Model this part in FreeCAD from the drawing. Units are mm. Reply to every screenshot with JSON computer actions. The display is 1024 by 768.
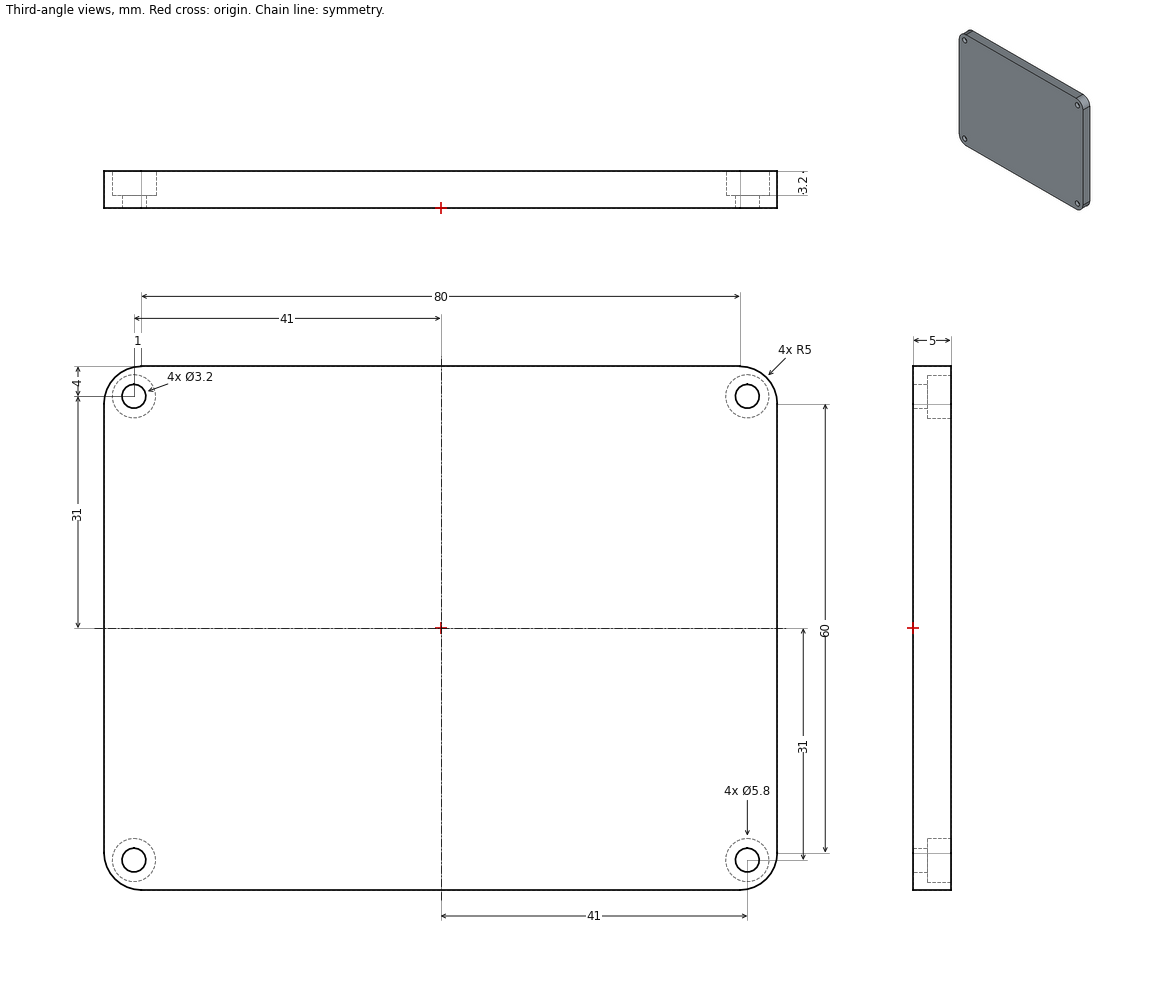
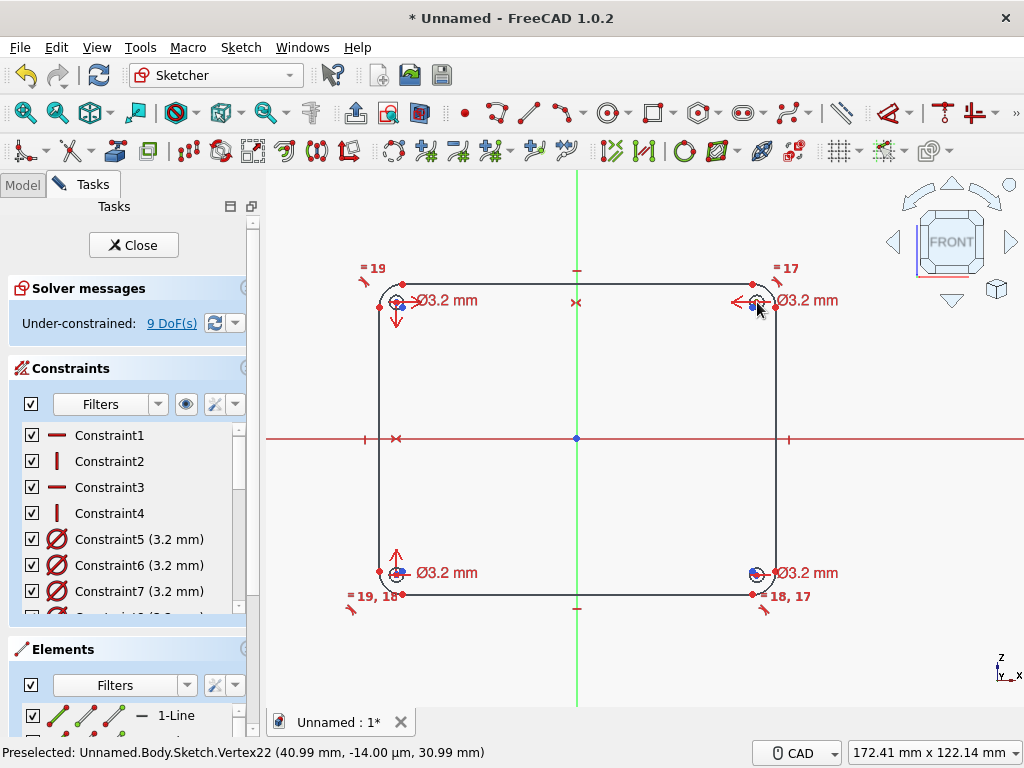
{"action": "scroll", "coordinate": [757, 575], "scroll_direction": "up", "scroll_amount": 4}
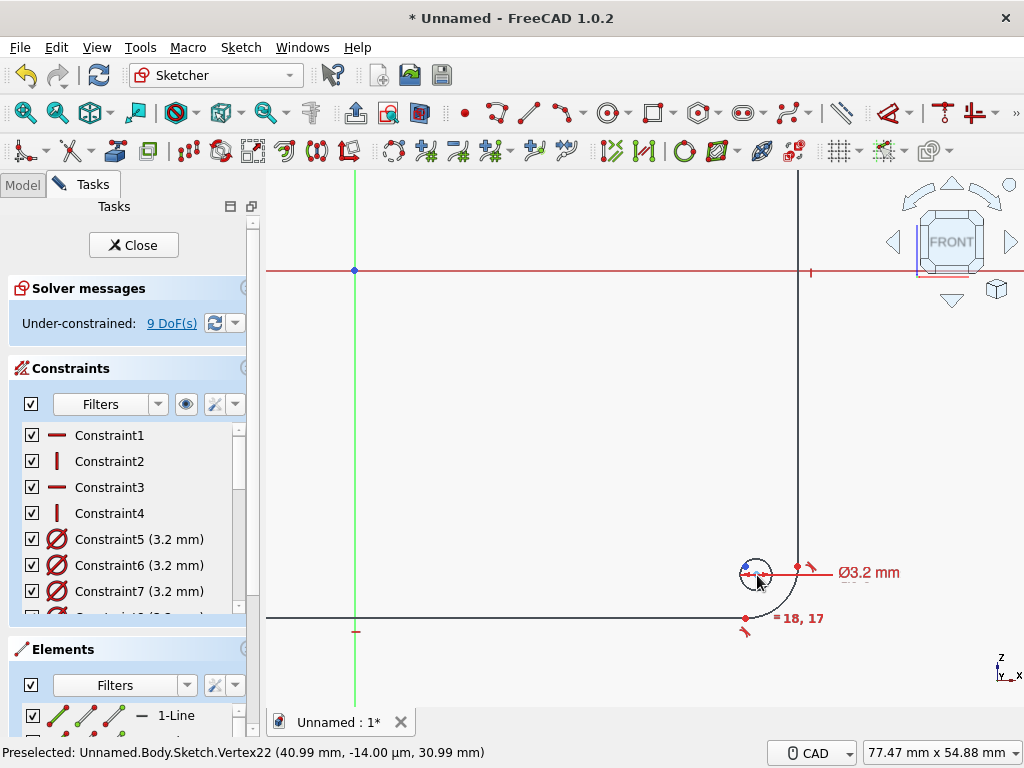
{"action": "left_click", "coordinate": [756, 575]}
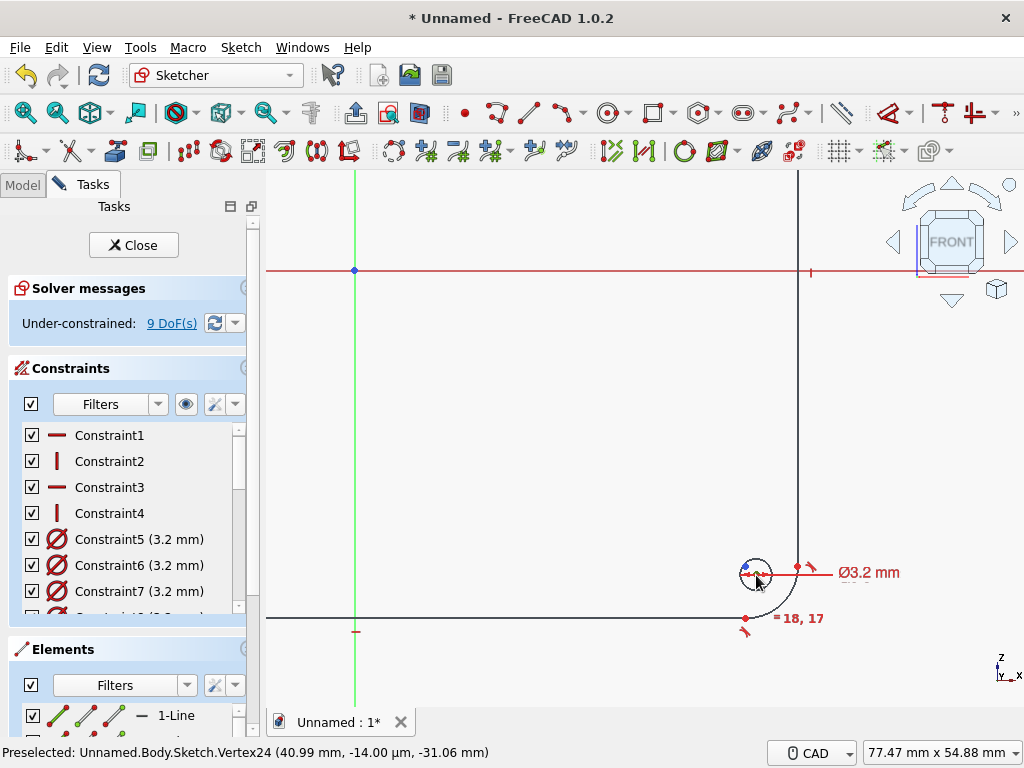
{"action": "left_click", "coordinate": [415, 271]}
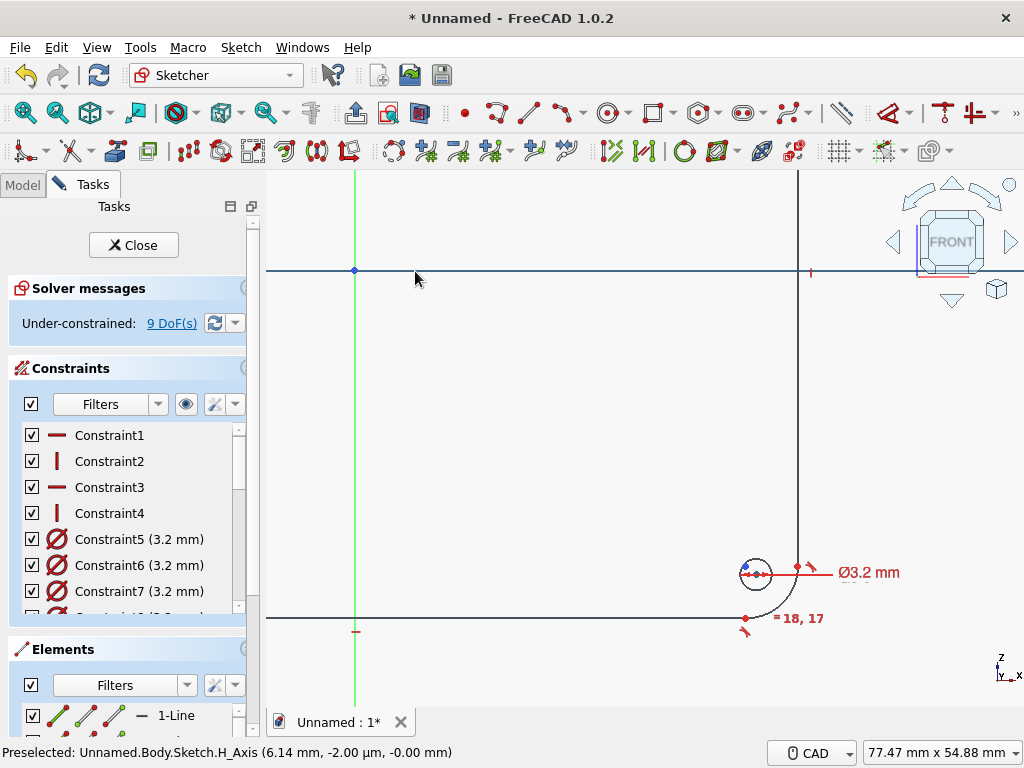
{"action": "key", "text": "s"}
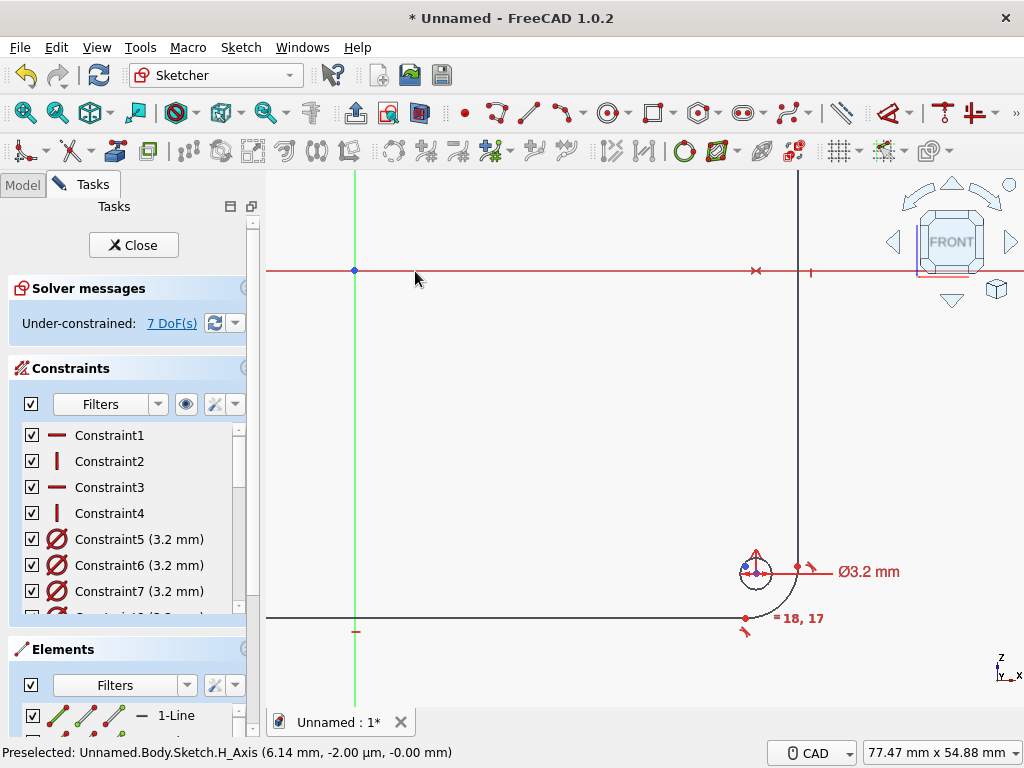
{"action": "scroll", "coordinate": [757, 575], "scroll_direction": "down", "scroll_amount": 4}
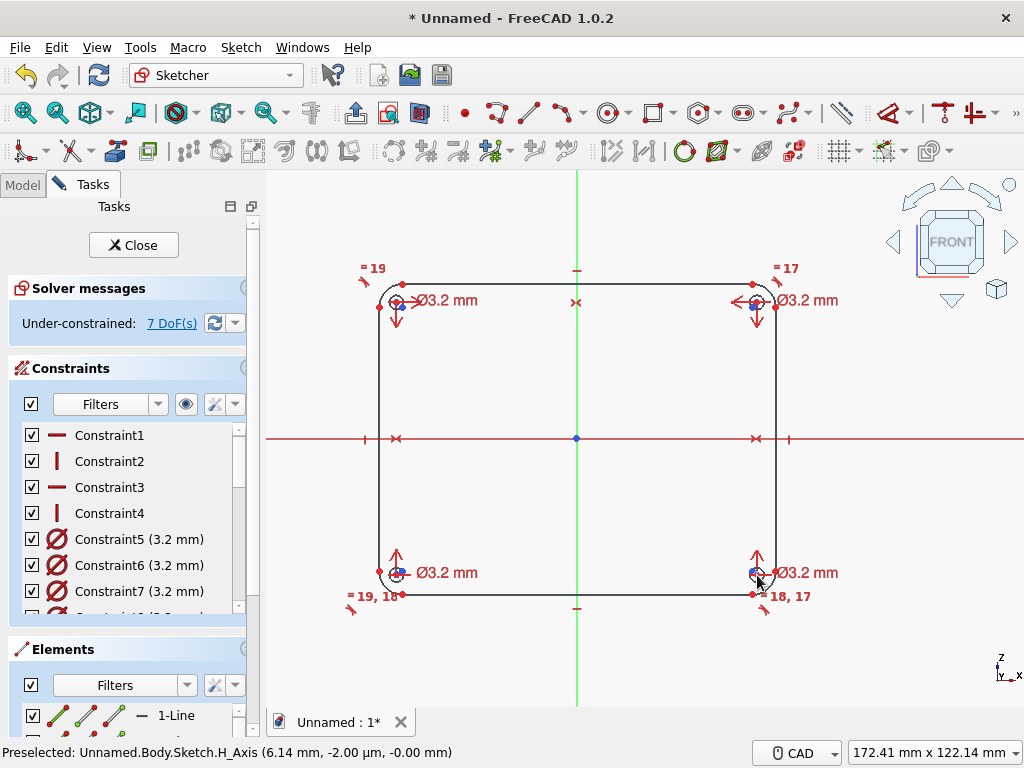
{"action": "scroll", "coordinate": [773, 297], "scroll_direction": "up", "scroll_amount": 3}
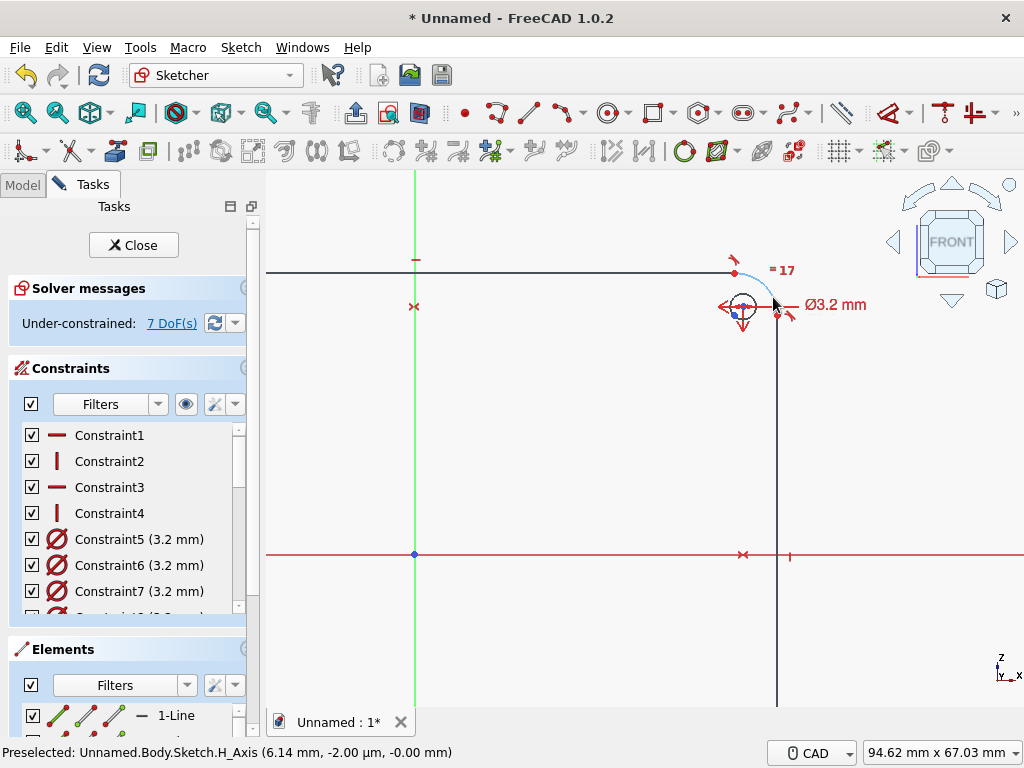
{"action": "left_click", "coordinate": [773, 297]}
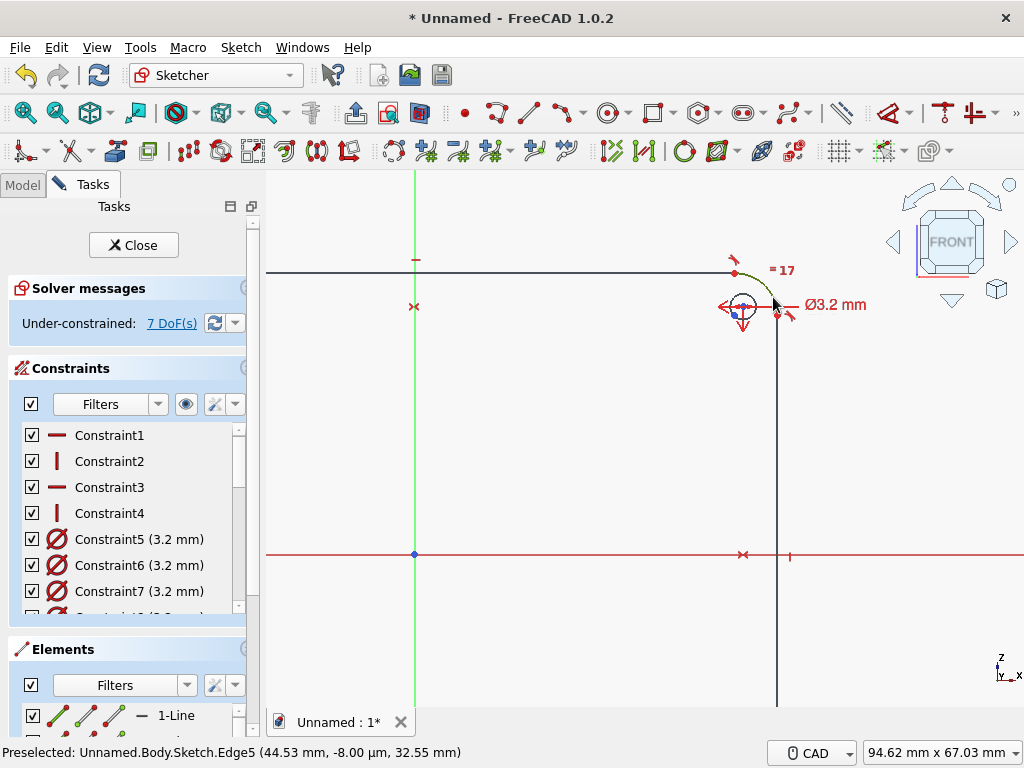
{"action": "key", "text": "k r"}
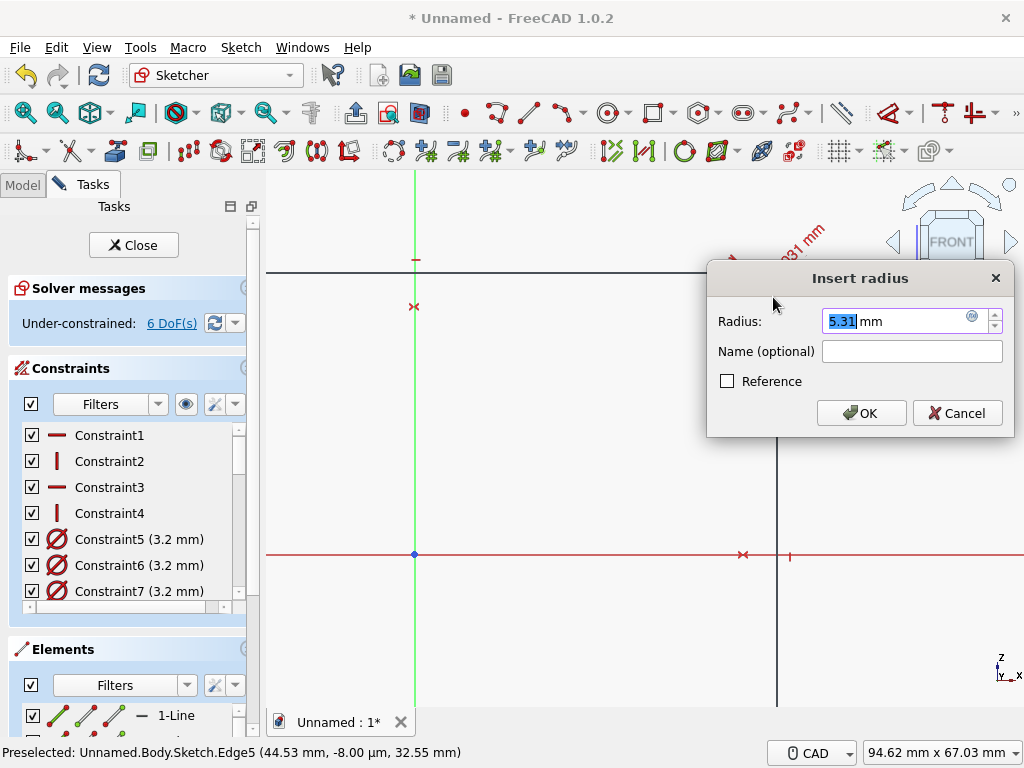
{"action": "type", "text": "5"}
{"action": "key", "text": "Return"}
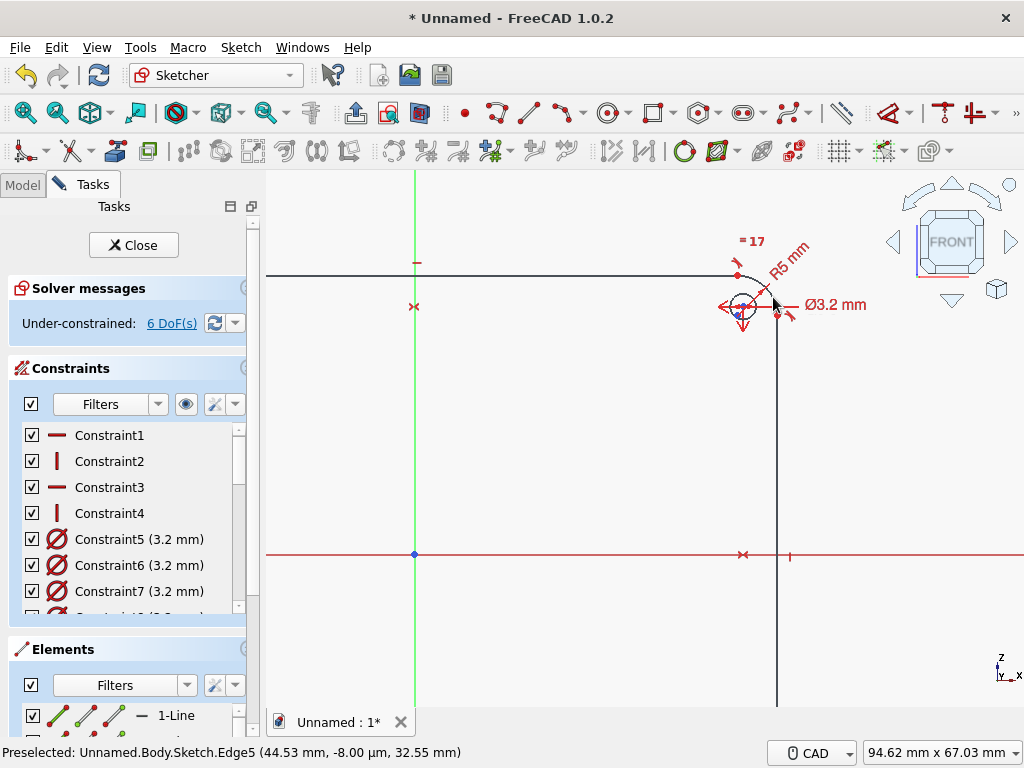
{"action": "left_click", "coordinate": [545, 276]}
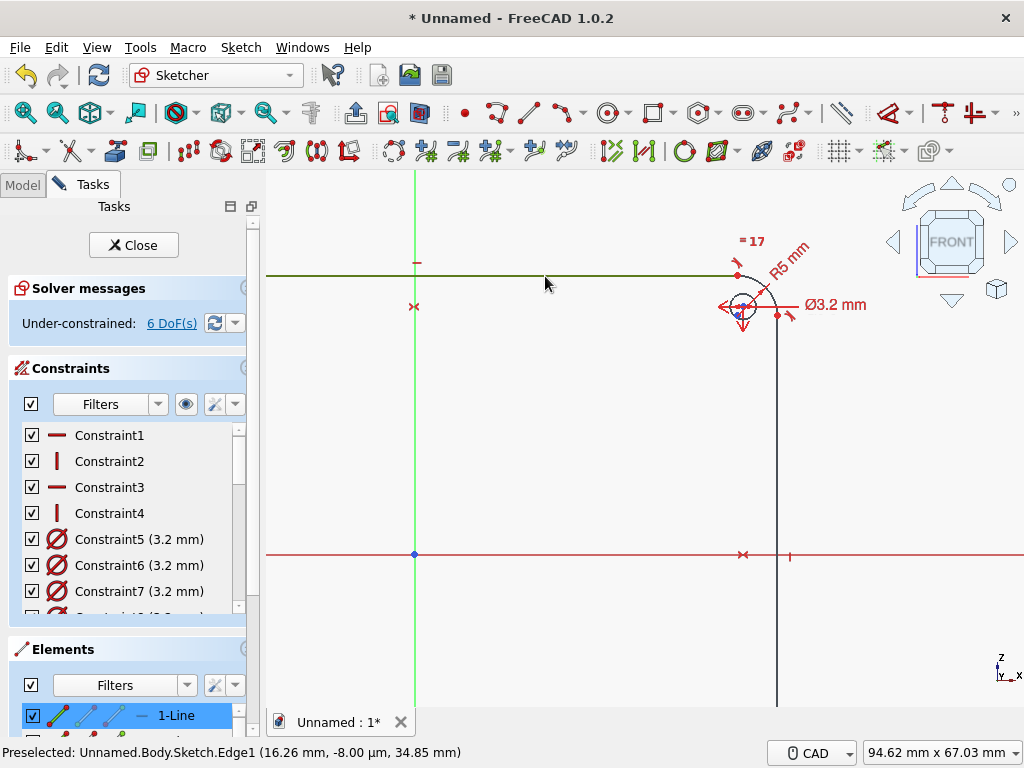
{"action": "key", "text": "l"}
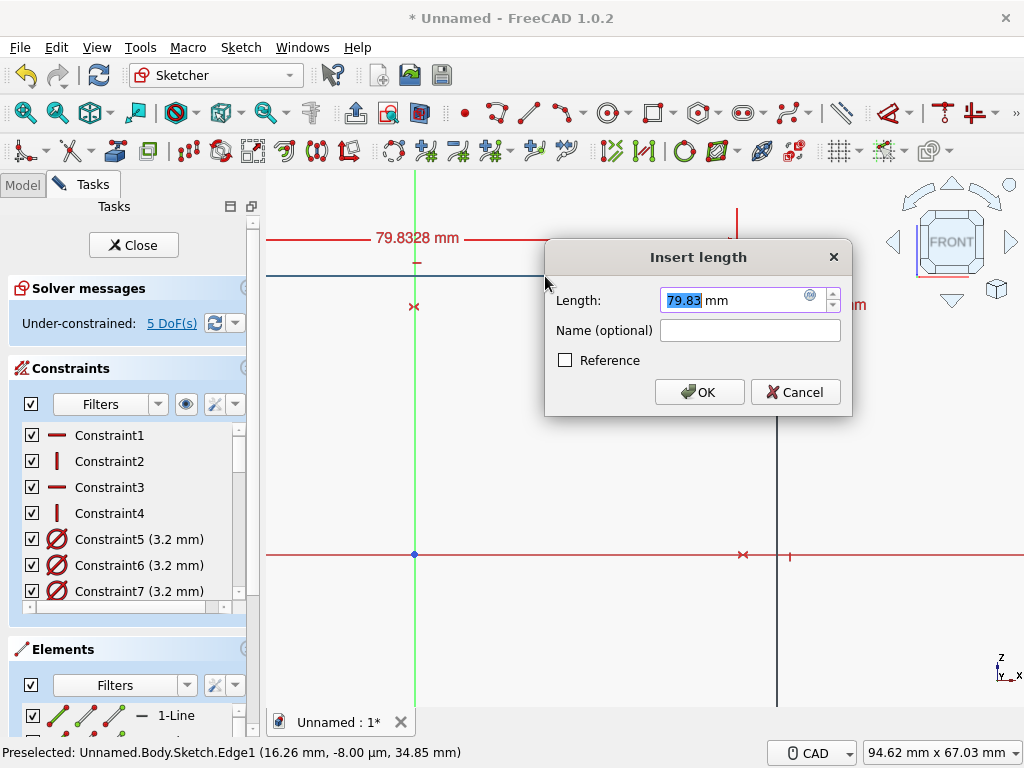
{"action": "type", "text": "80"}
{"action": "key", "text": "Return"}